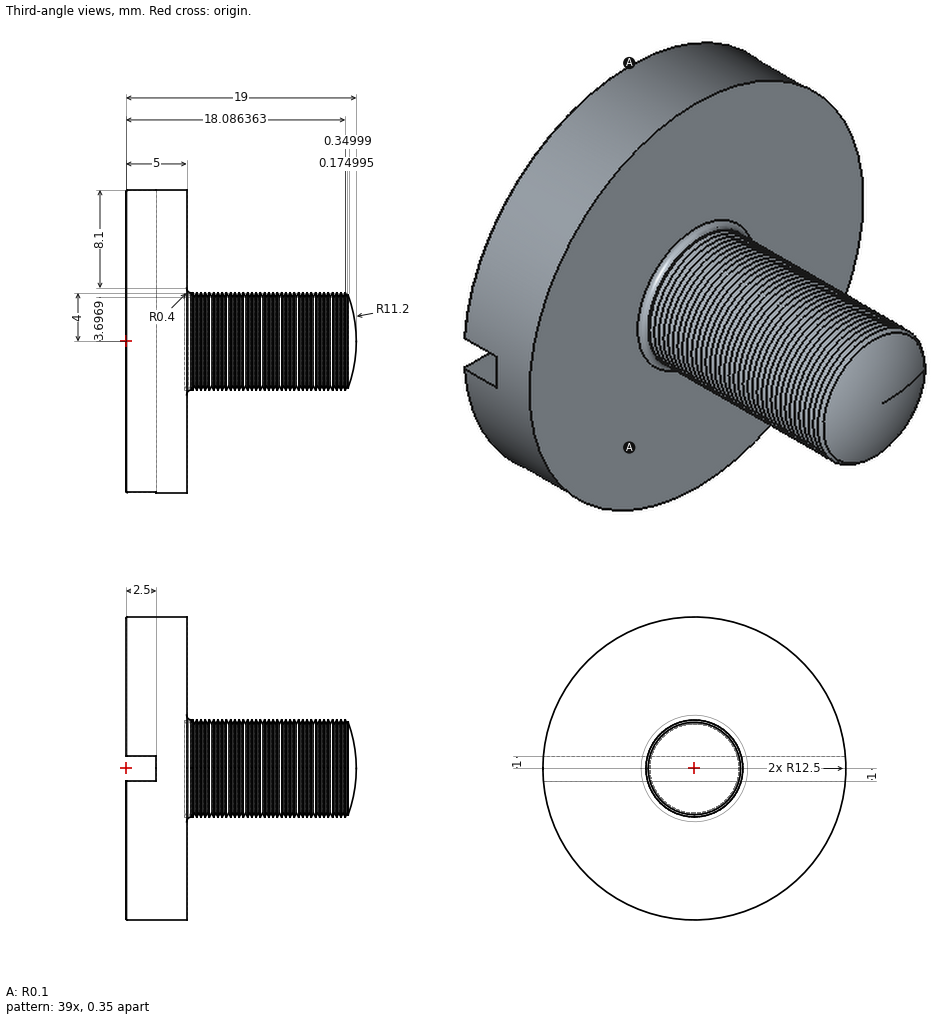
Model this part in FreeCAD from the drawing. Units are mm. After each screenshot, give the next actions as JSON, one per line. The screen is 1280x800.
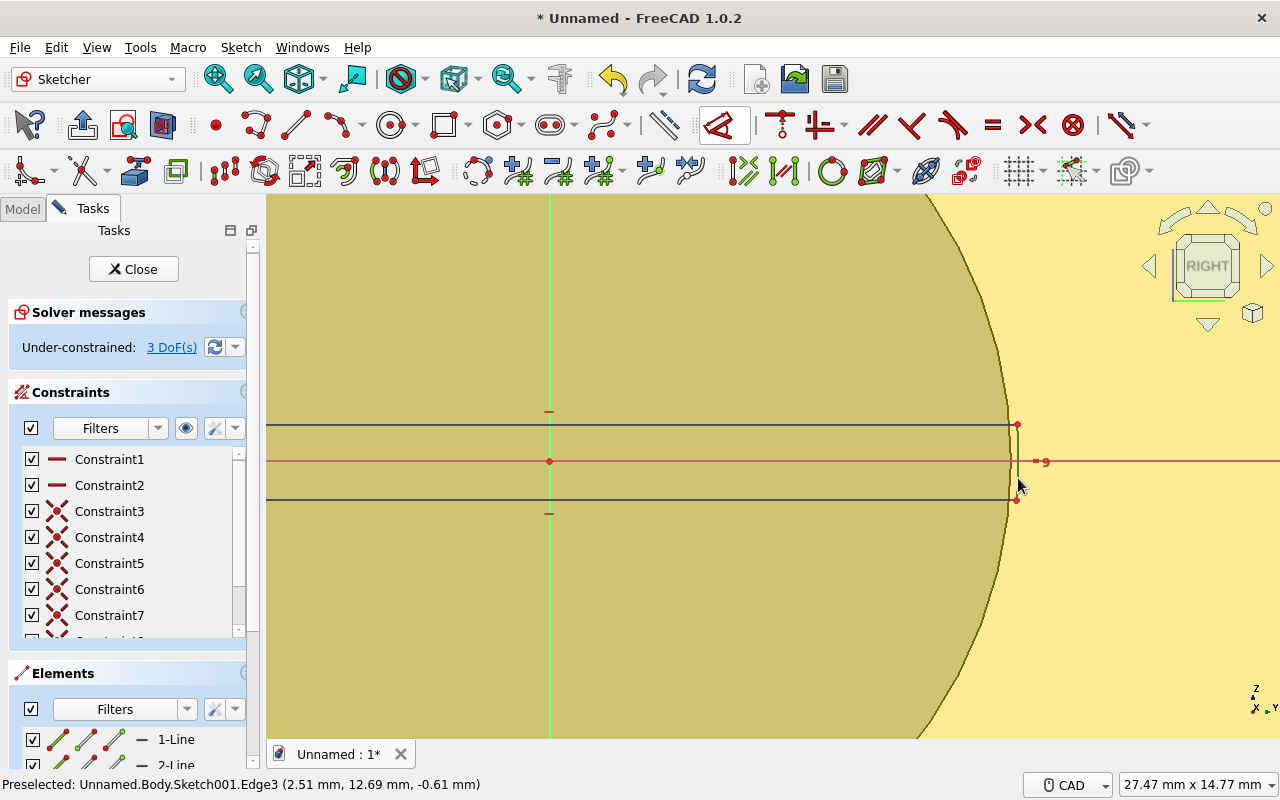
{"action": "left_click", "coordinate": [744, 126]}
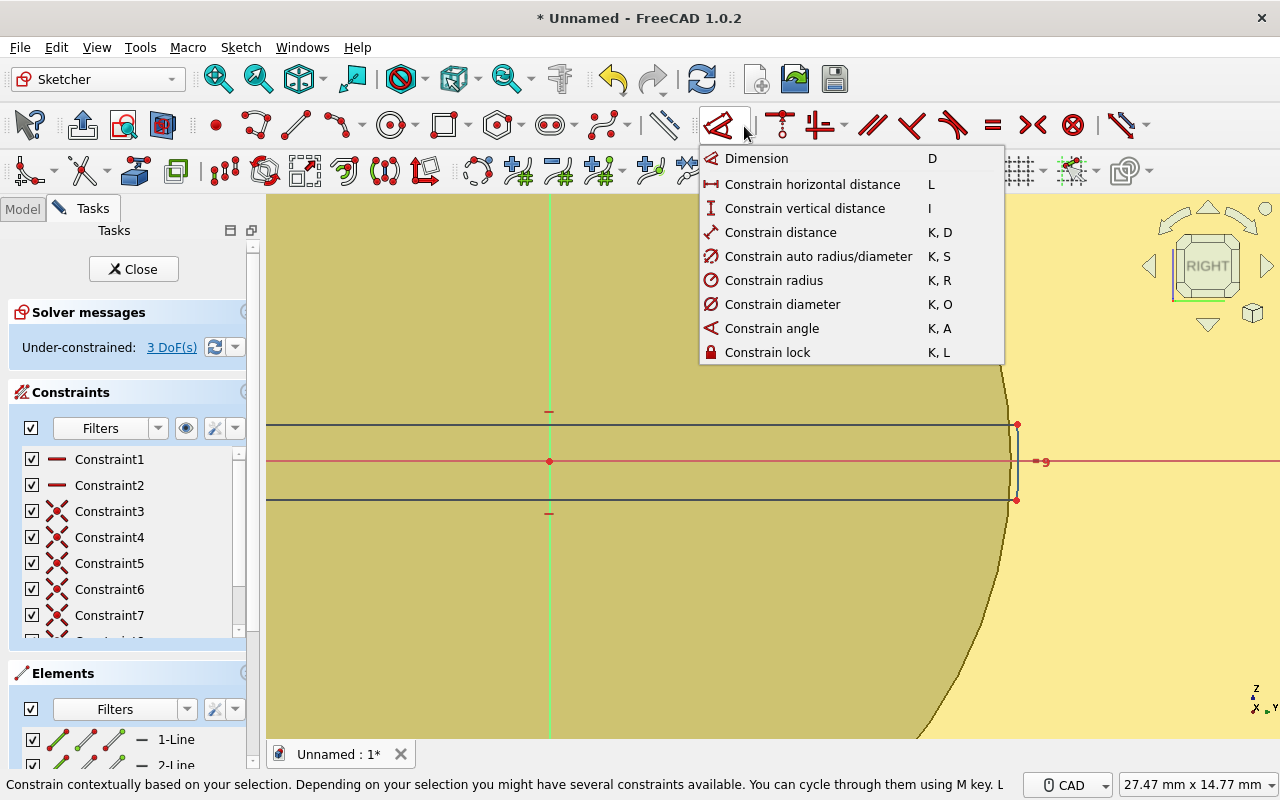
{"action": "left_click", "coordinate": [852, 280]}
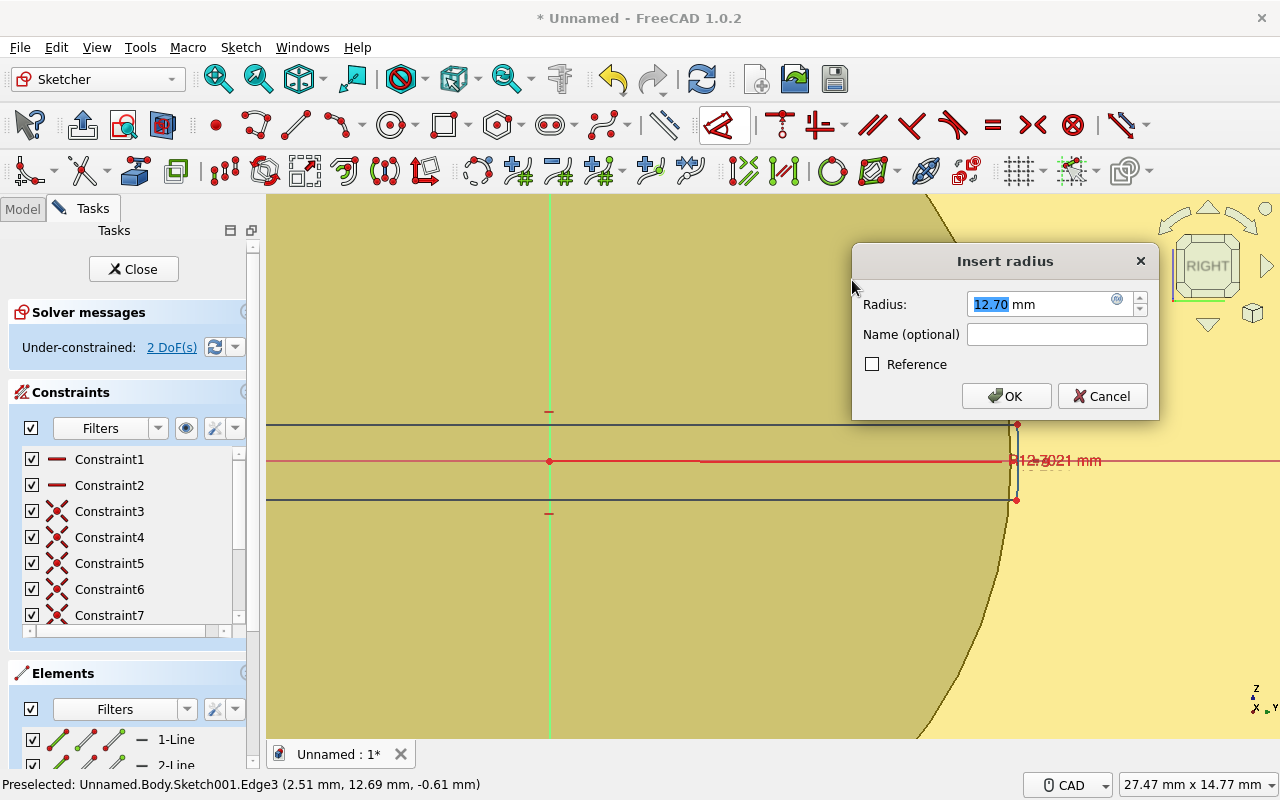
{"action": "type", "text": "12.5"}
{"action": "key", "text": "Return"}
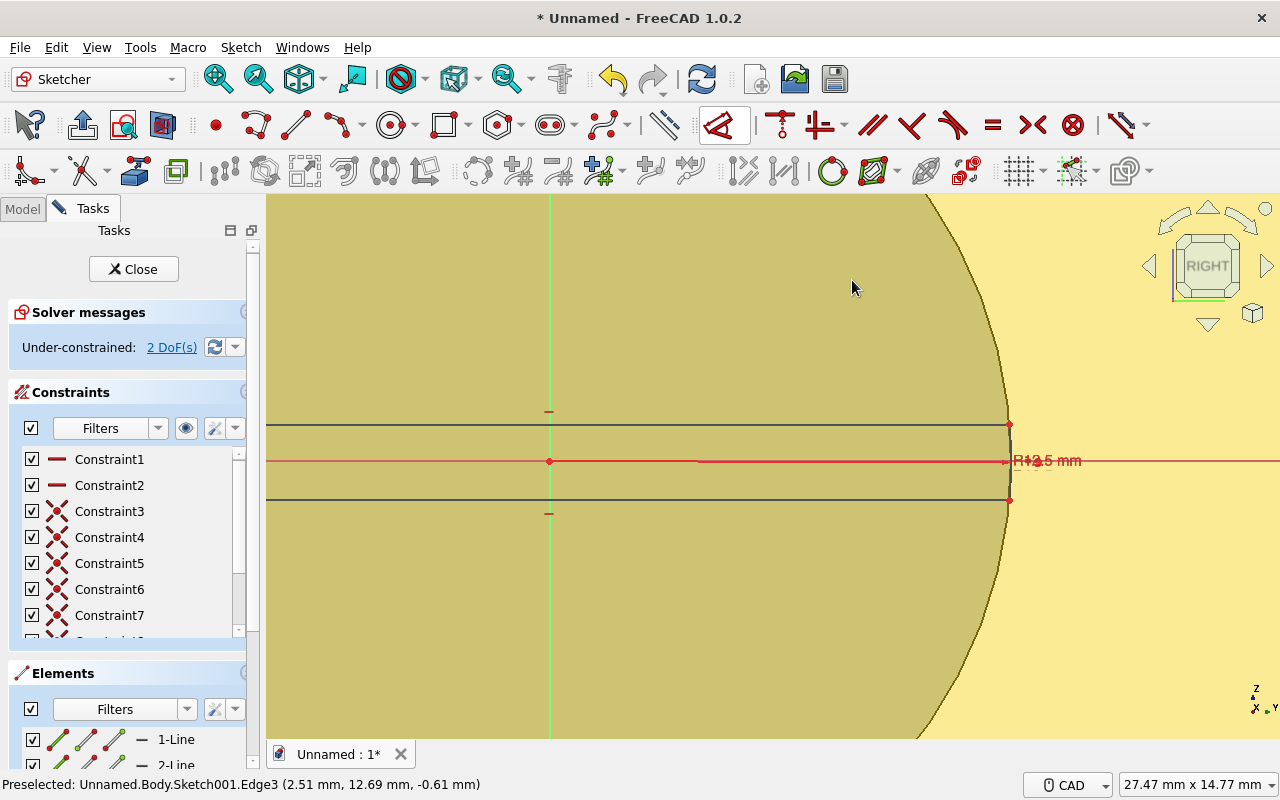
{"action": "scroll", "coordinate": [1019, 478], "scroll_direction": "down", "scroll_amount": 2}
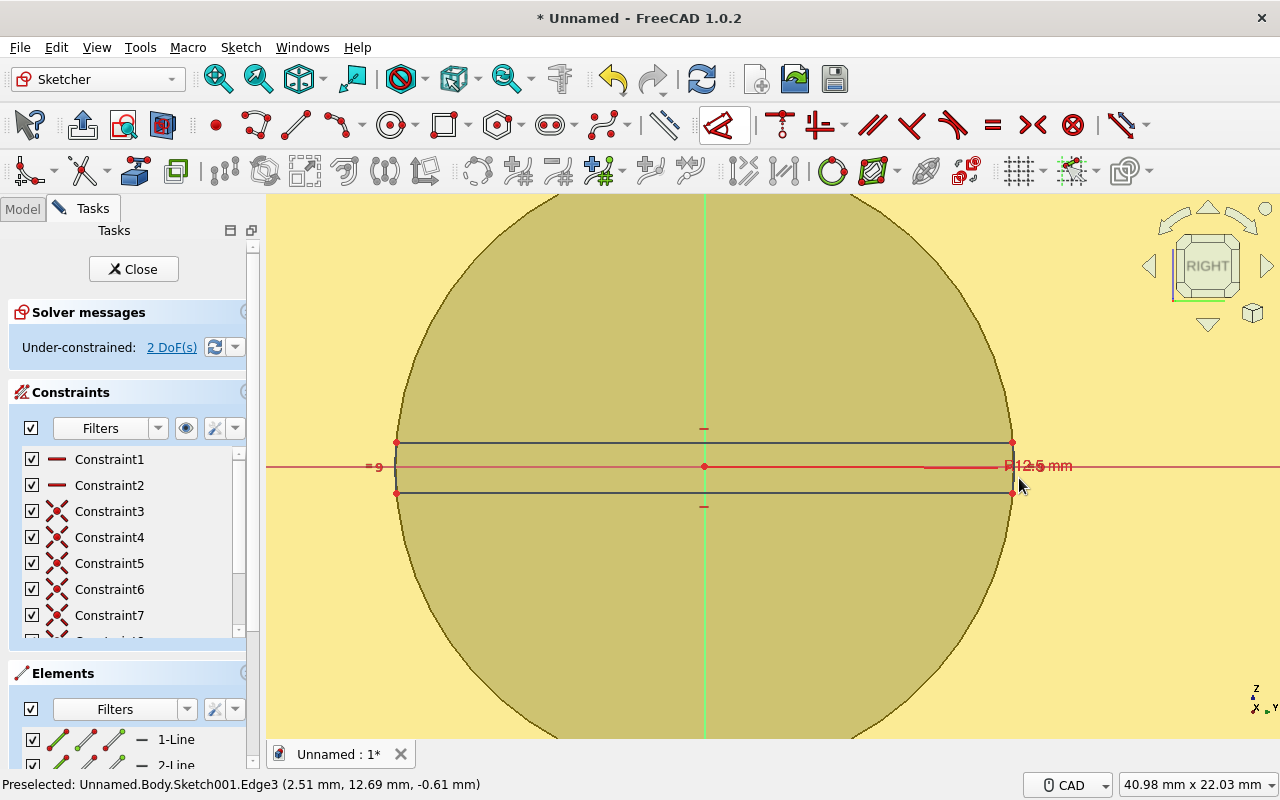
{"action": "scroll", "coordinate": [396, 443], "scroll_direction": "up", "scroll_amount": 3}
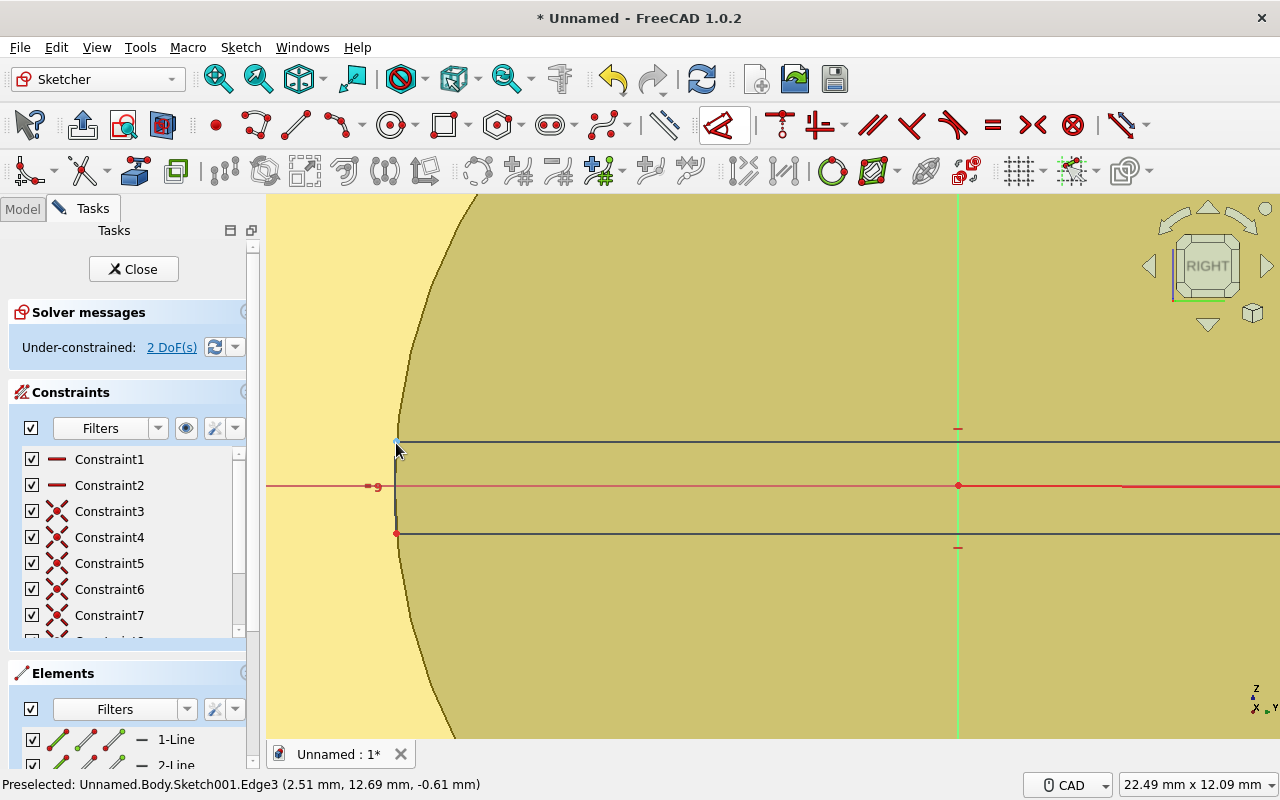
{"action": "left_click", "coordinate": [396, 442]}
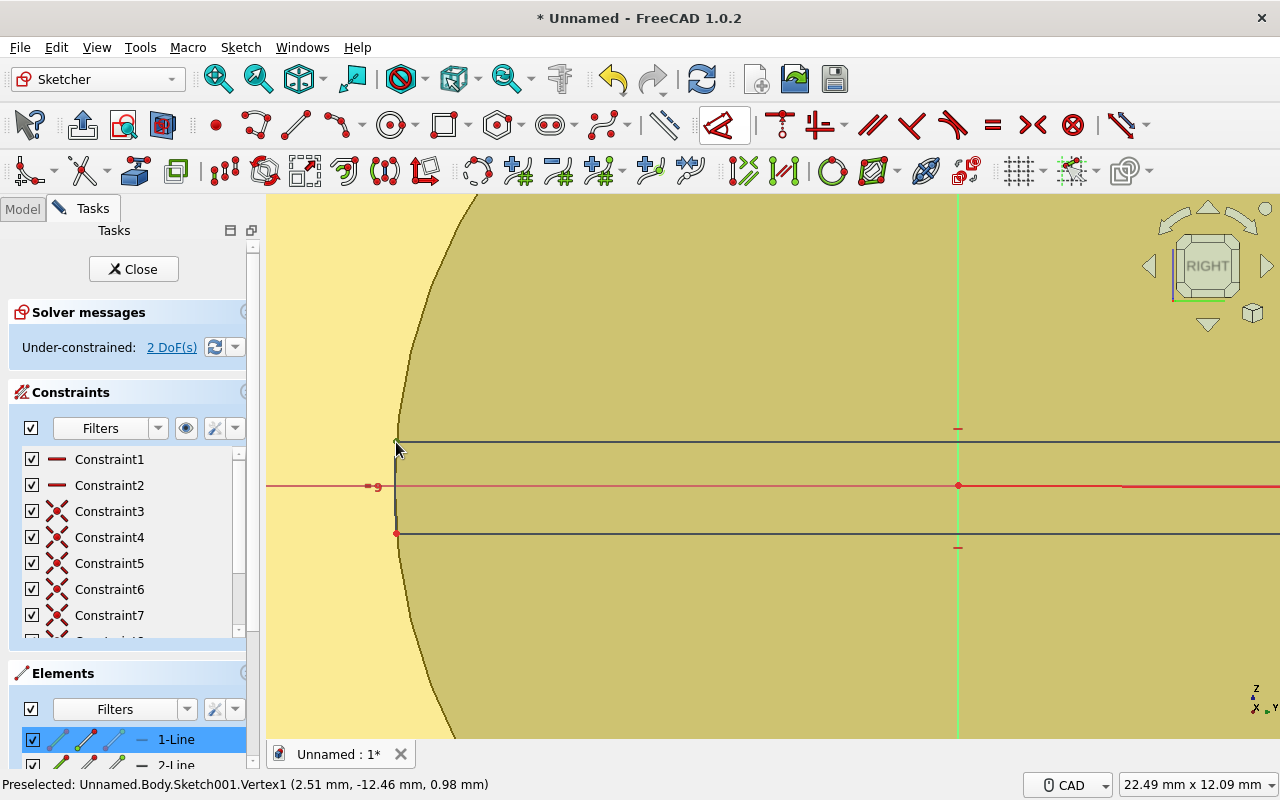
{"action": "left_click", "coordinate": [744, 126]}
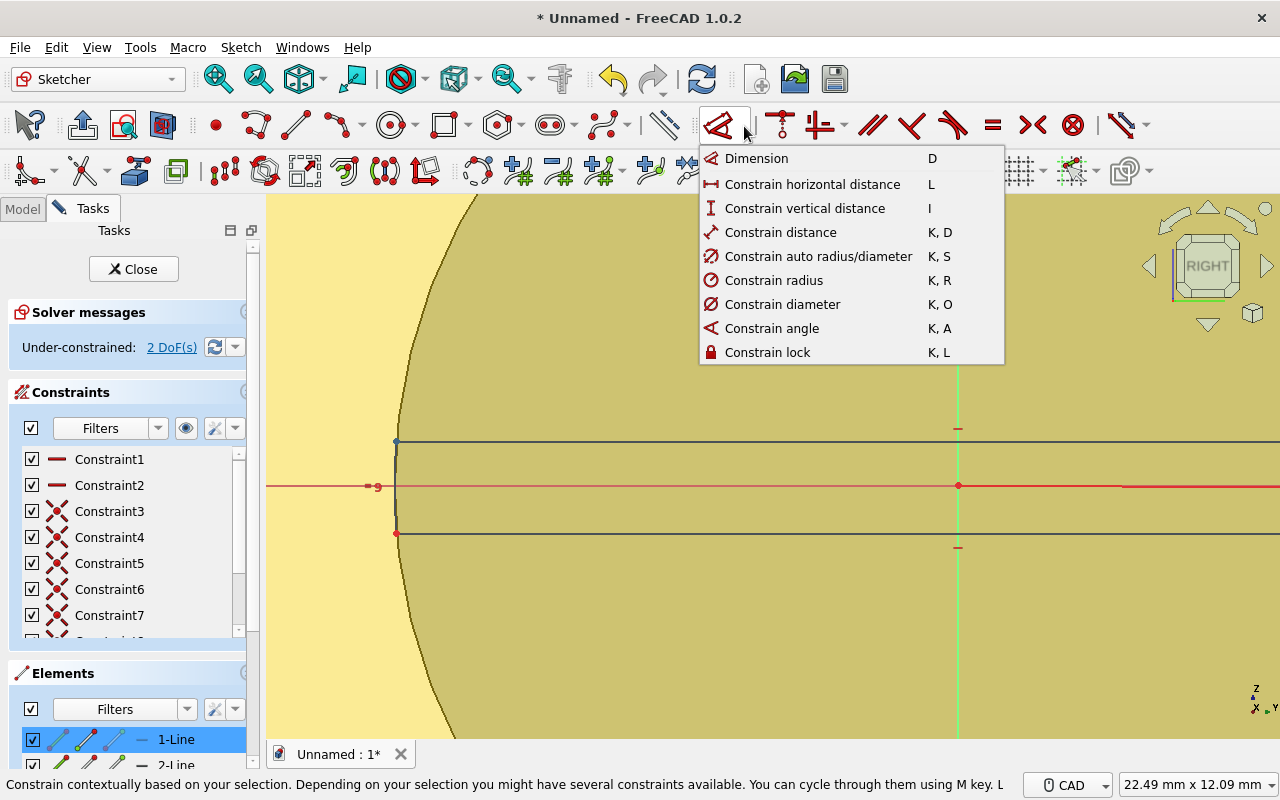
{"action": "left_click", "coordinate": [852, 208]}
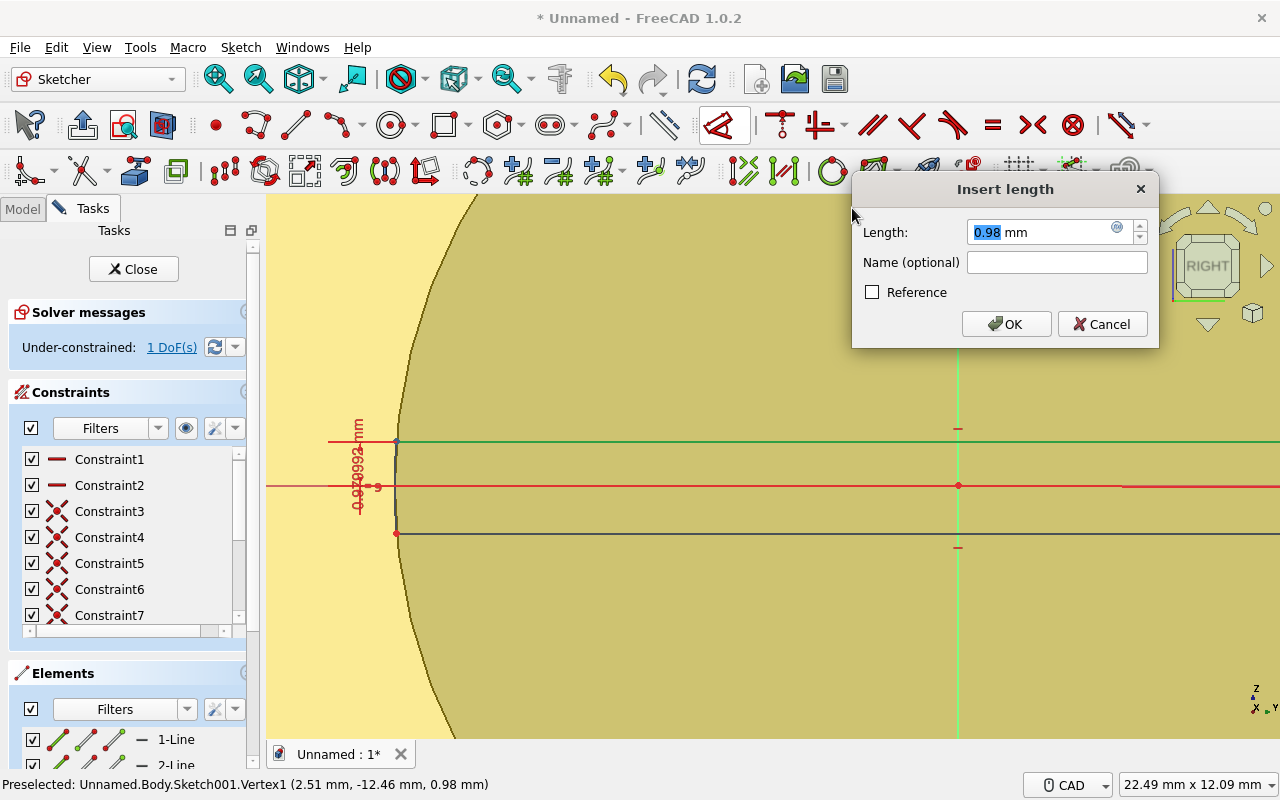
{"action": "type", "text": "1"}
{"action": "key", "text": "Return"}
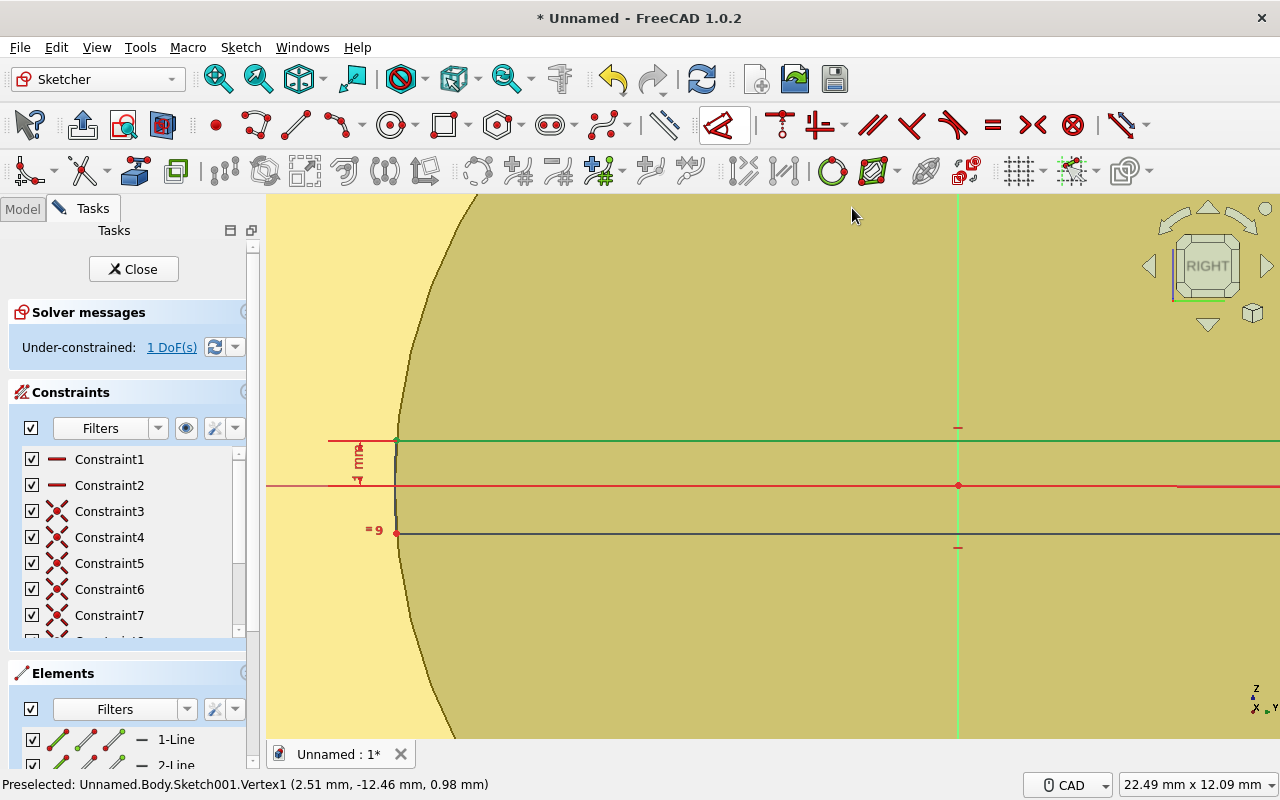
{"action": "scroll", "coordinate": [396, 443], "scroll_direction": "down", "scroll_amount": 3}